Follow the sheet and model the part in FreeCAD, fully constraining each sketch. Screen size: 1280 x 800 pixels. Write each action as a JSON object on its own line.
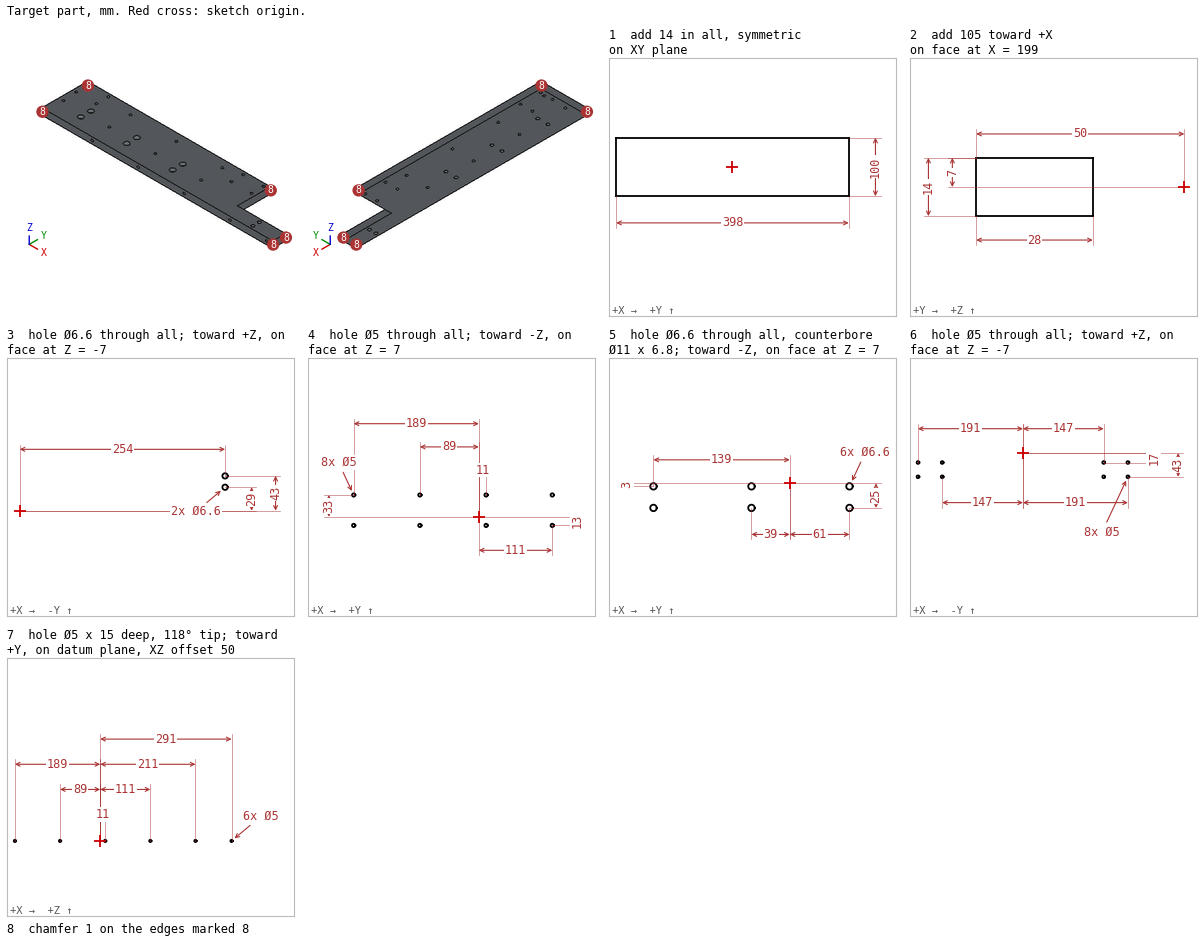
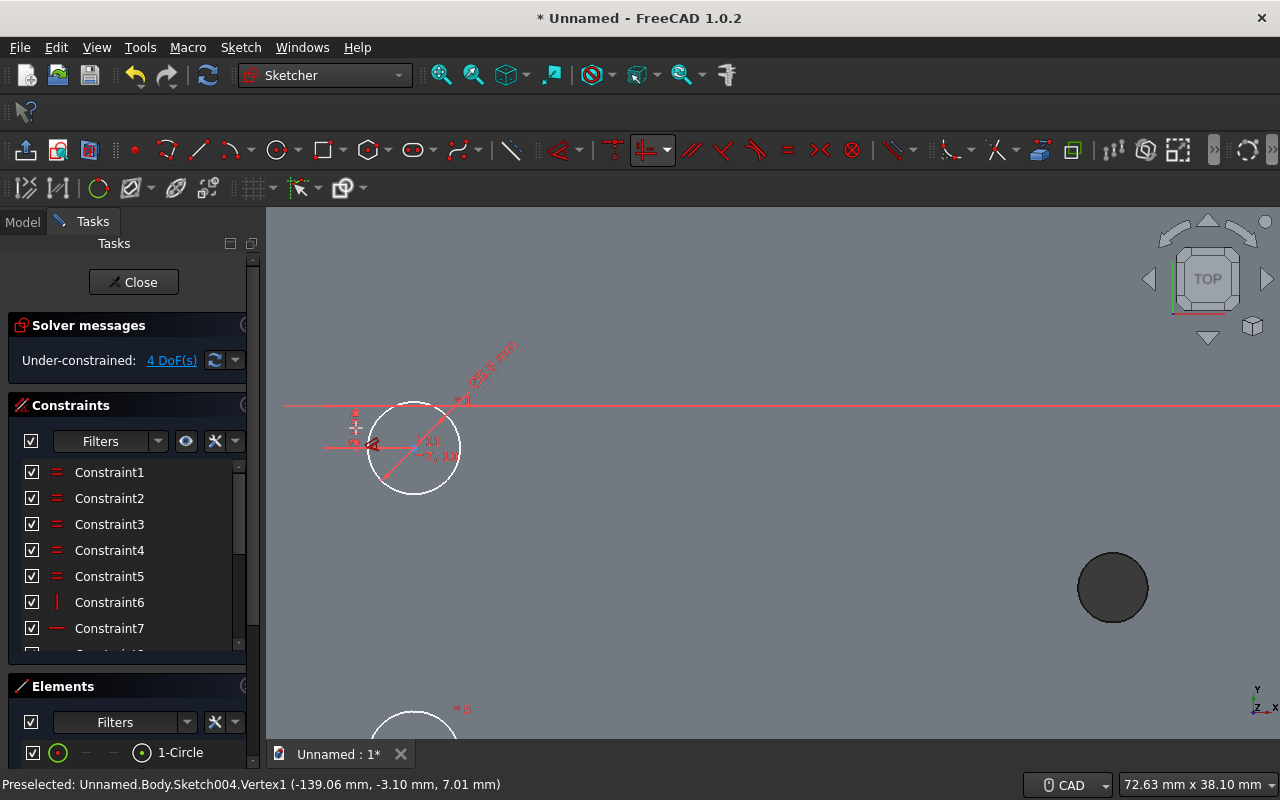
{"action": "scroll", "coordinate": [425, 440], "scroll_direction": "down", "scroll_amount": 8}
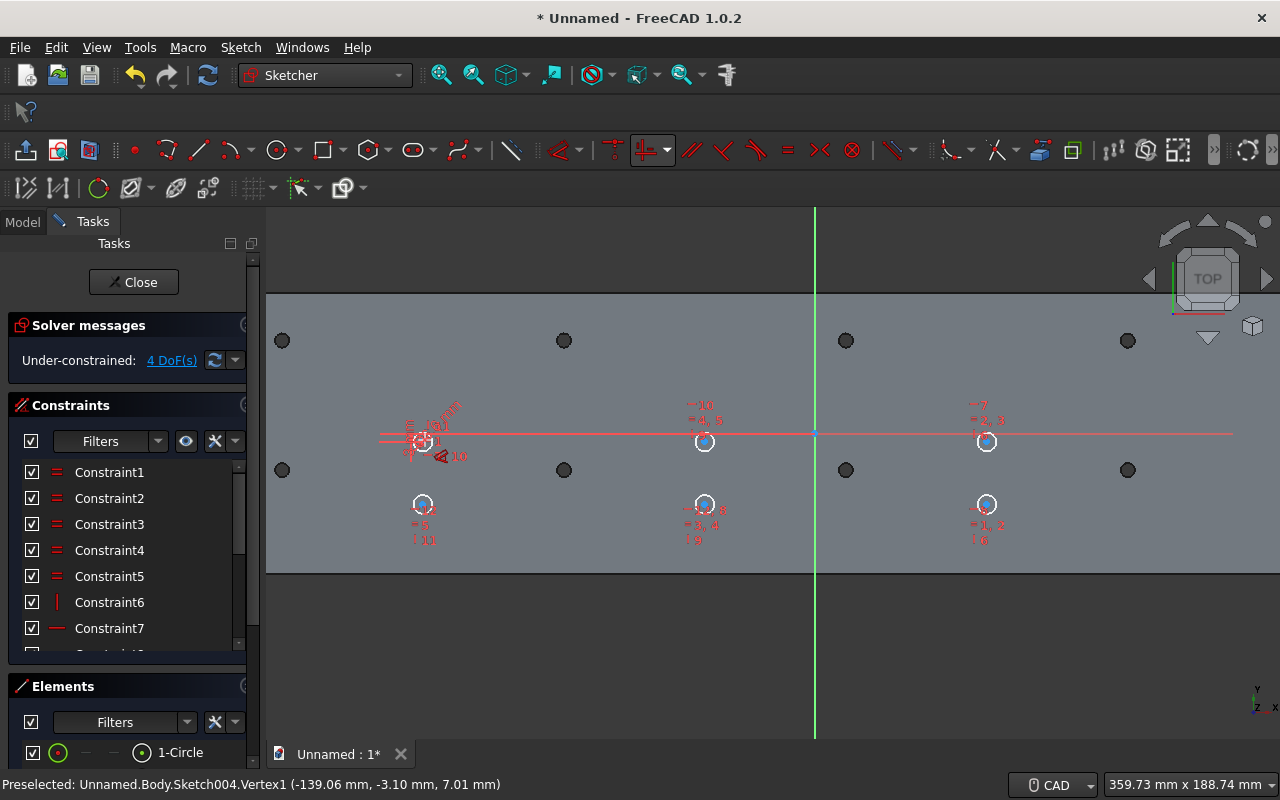
{"action": "left_click", "coordinate": [987, 504]}
{"action": "left_click", "coordinate": [901, 400]}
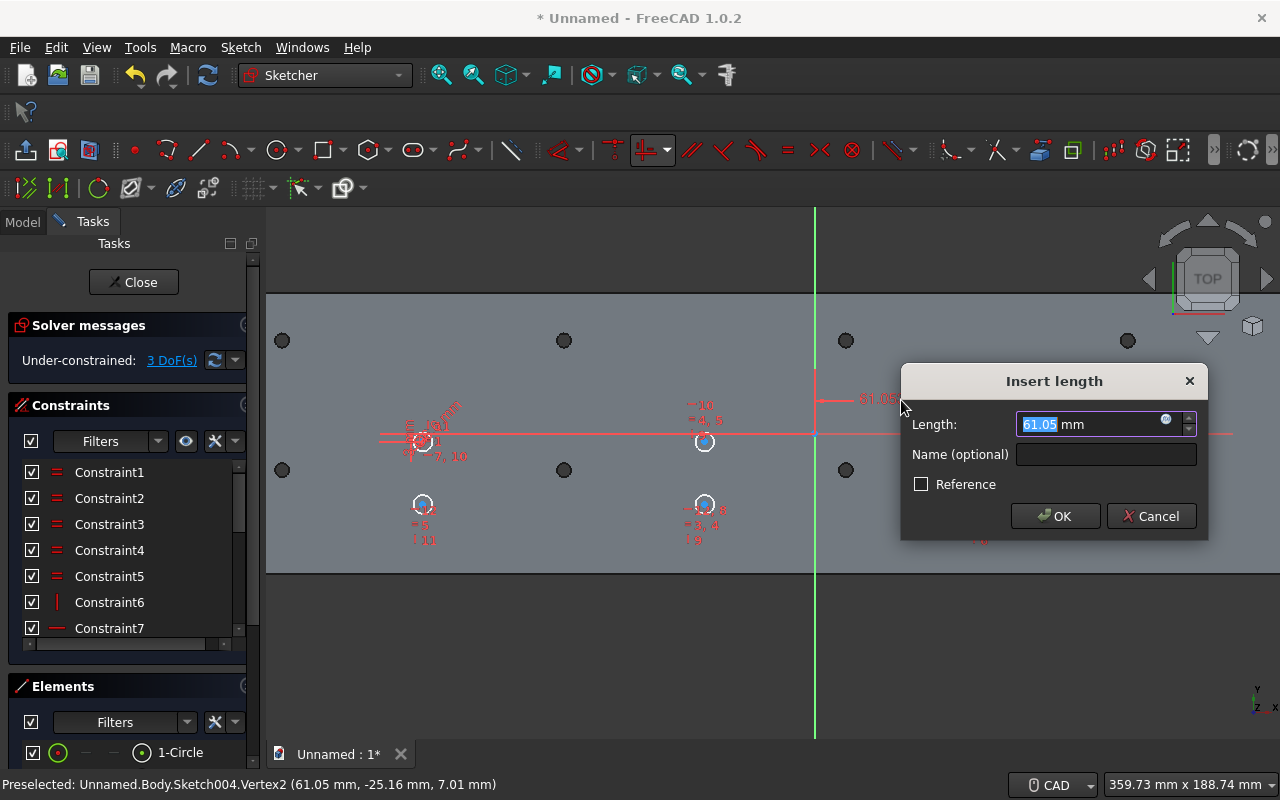
{"action": "type", "text": "61"}
{"action": "key", "text": "Return"}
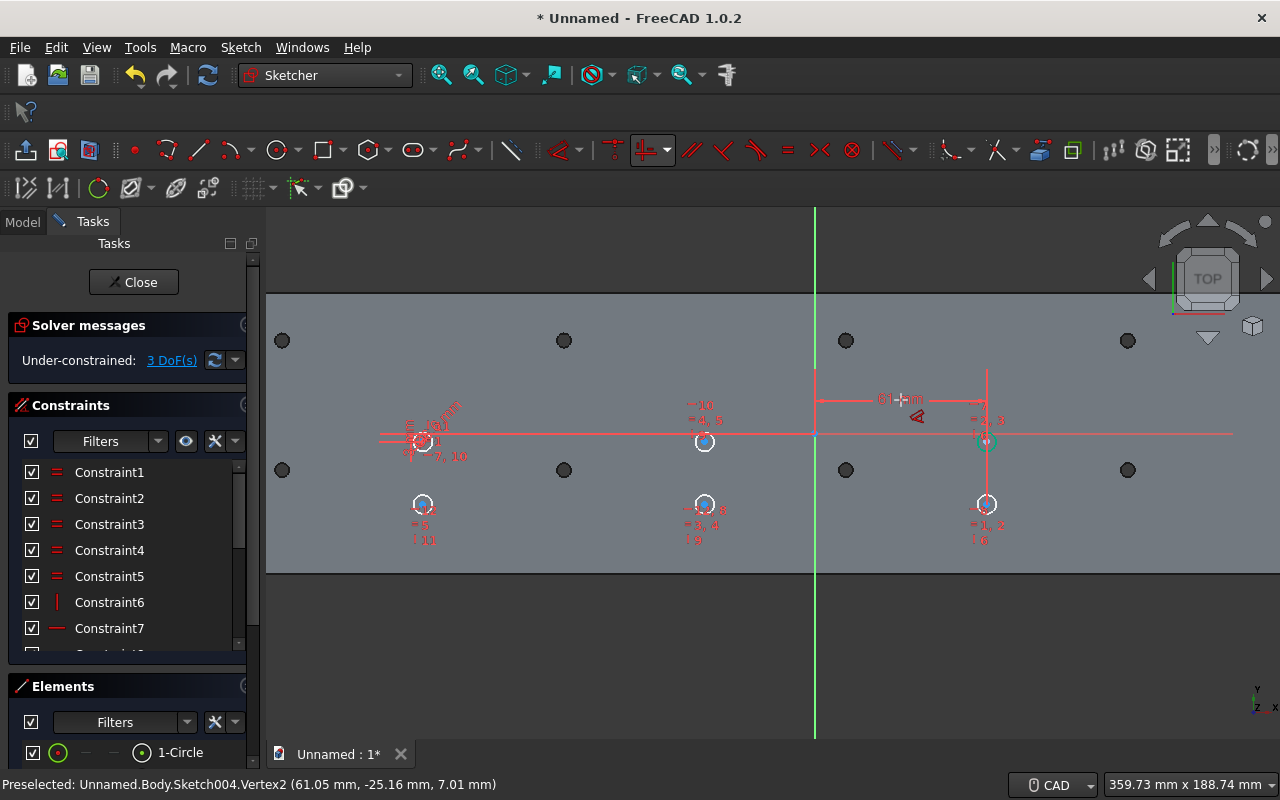
{"action": "left_click", "coordinate": [987, 504]}
{"action": "left_click", "coordinate": [1021, 469]}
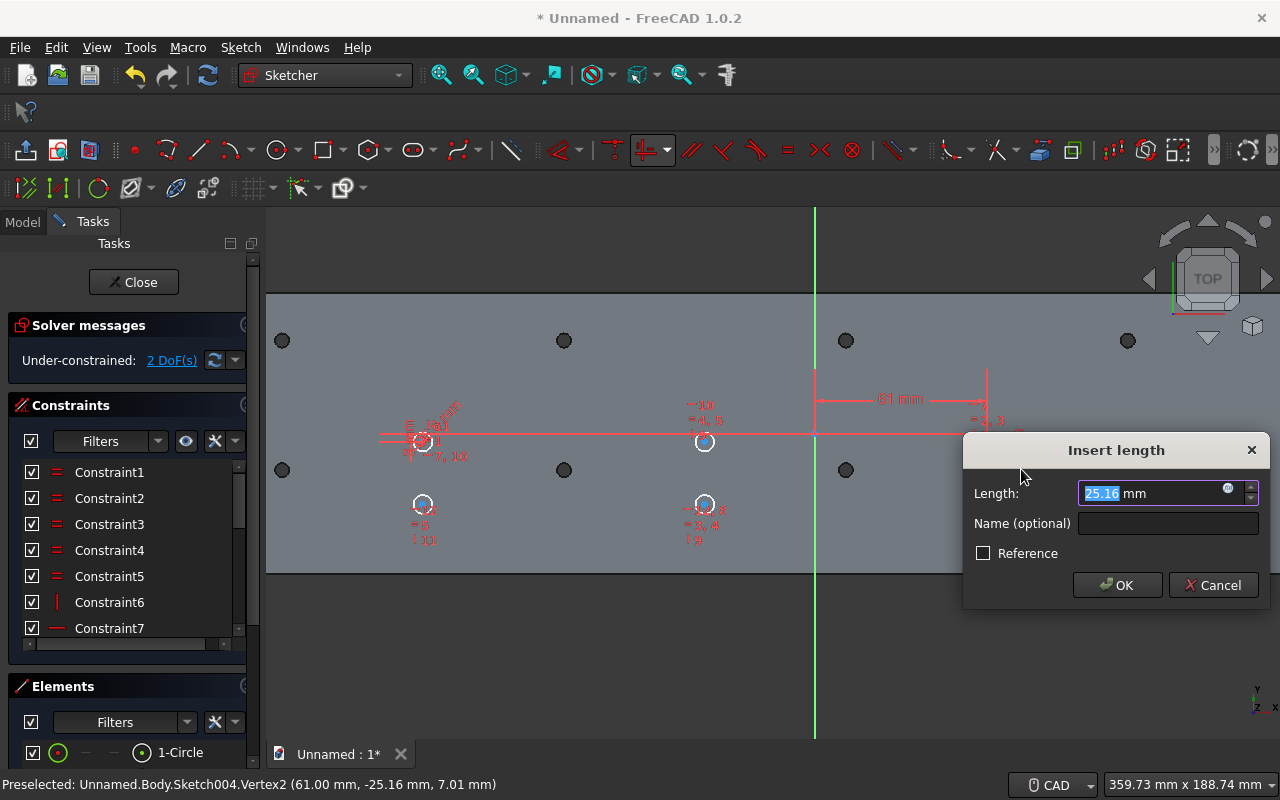
{"action": "type", "text": "25"}
{"action": "key", "text": "Return"}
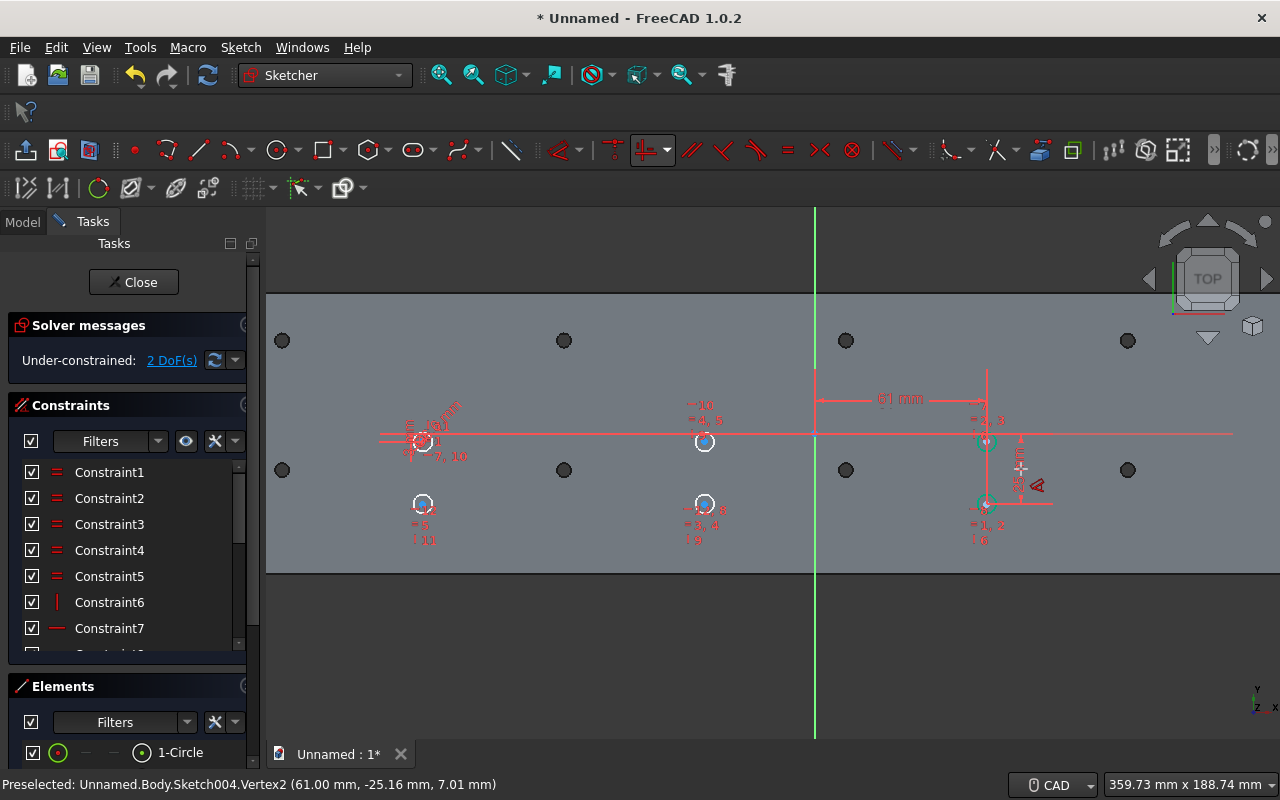
{"action": "left_click", "coordinate": [705, 504]}
{"action": "left_click", "coordinate": [760, 400]}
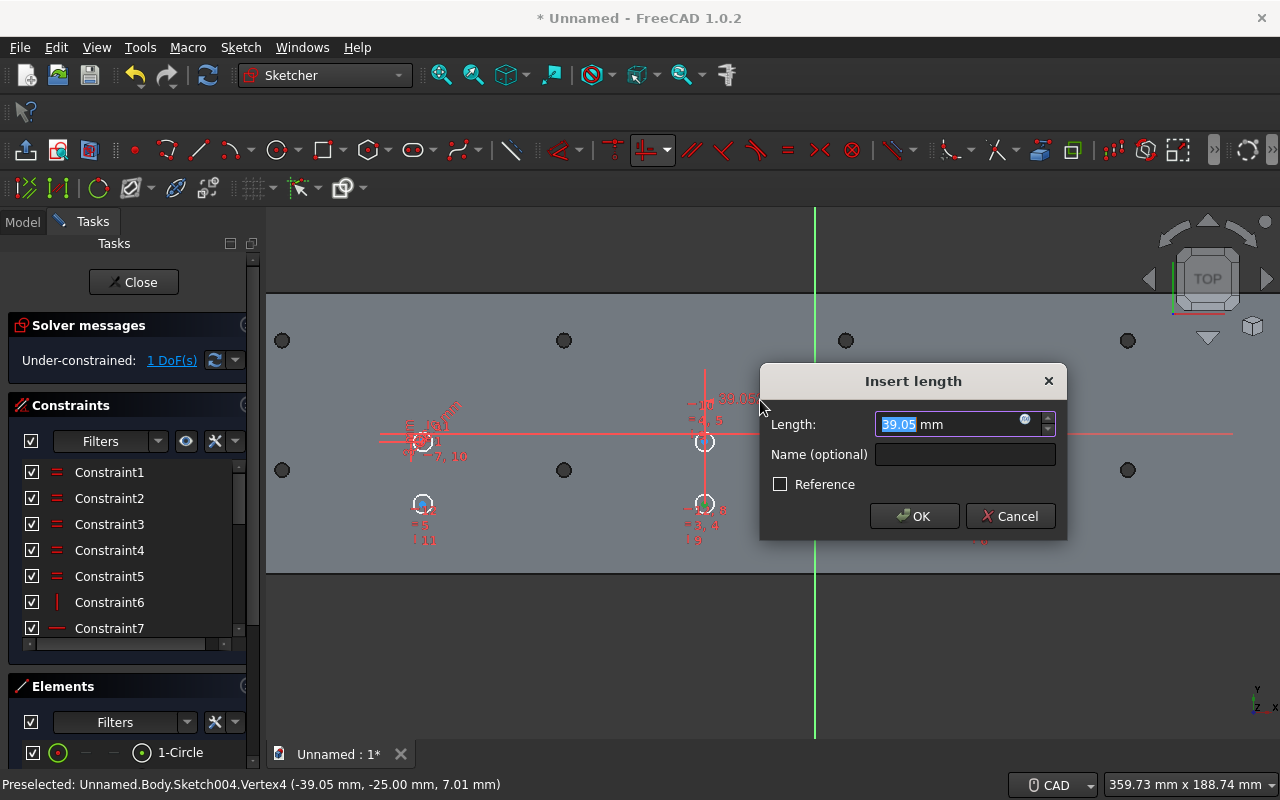
{"action": "type", "text": "39"}
{"action": "key", "text": "Return"}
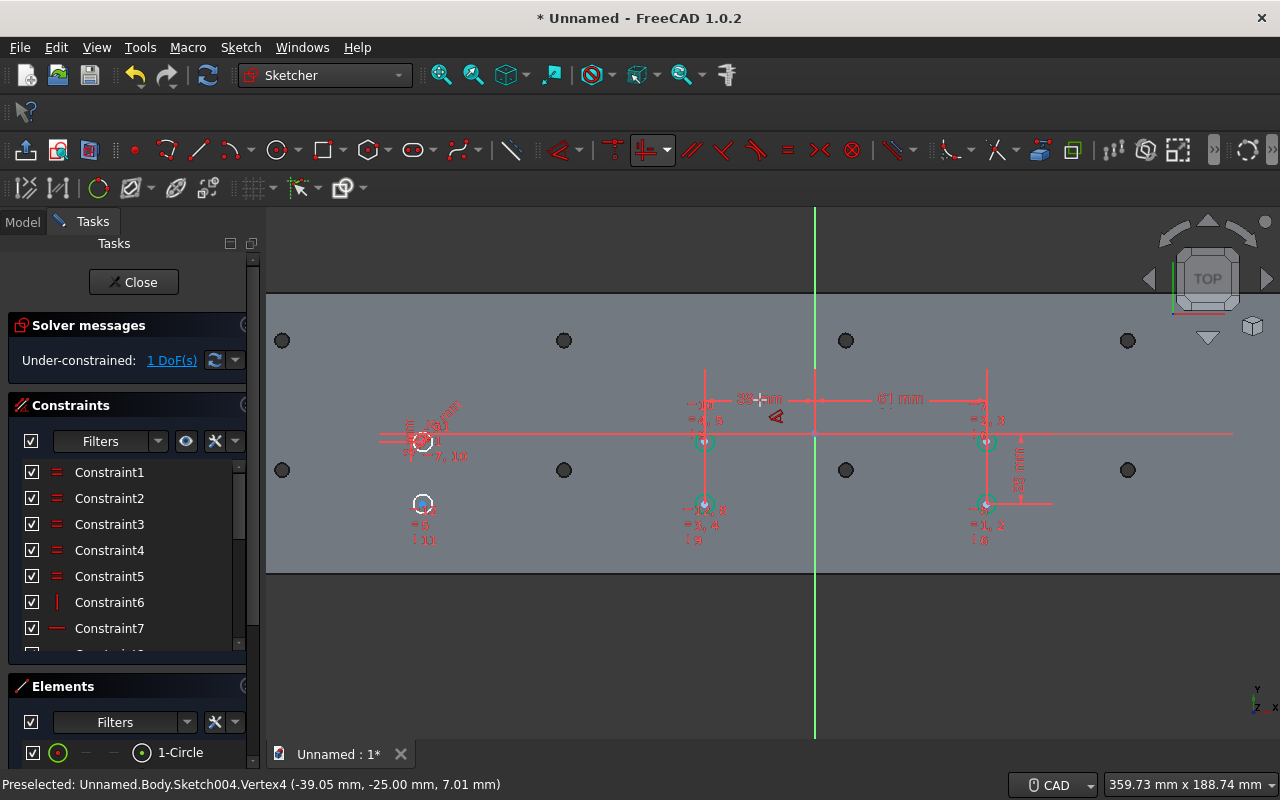
{"action": "left_click", "coordinate": [423, 442]}
{"action": "left_click", "coordinate": [619, 400]}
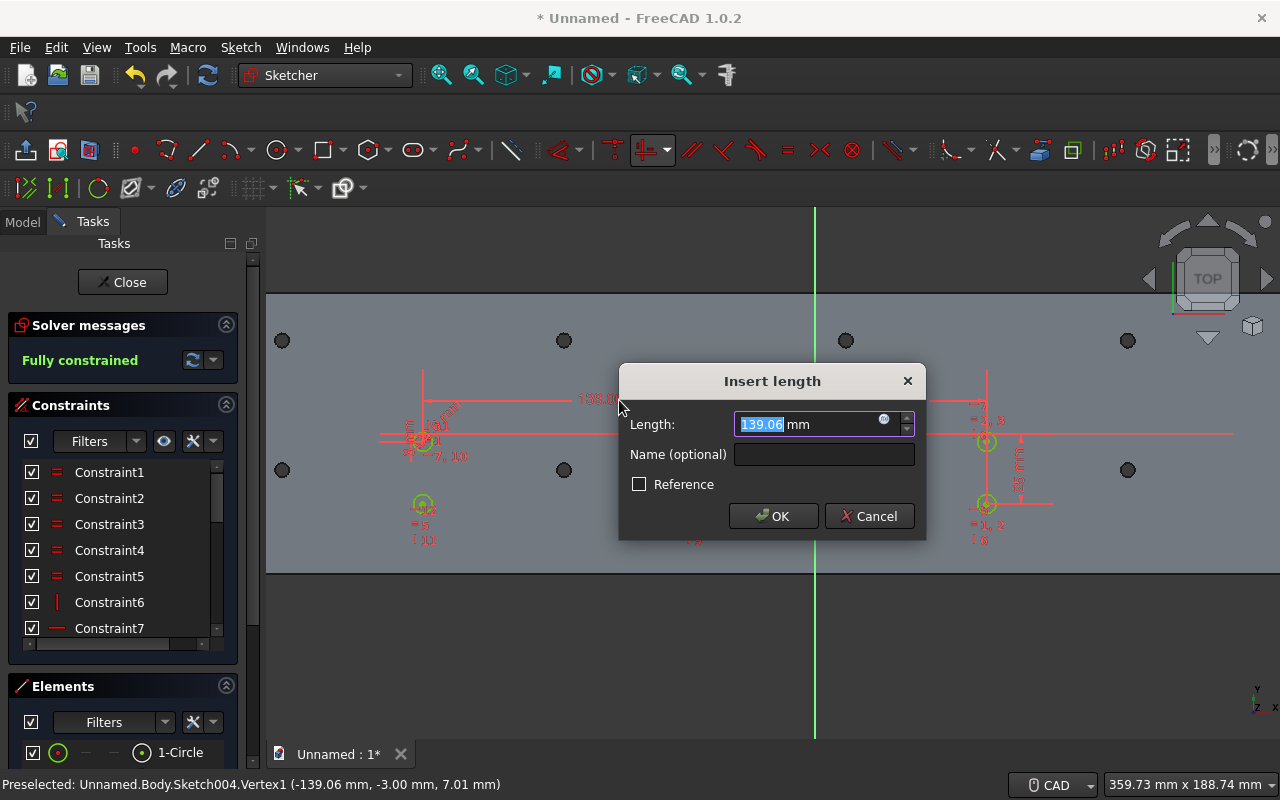
{"action": "type", "text": "139"}
{"action": "key", "text": "Return"}
{"action": "key", "text": "Escape"}